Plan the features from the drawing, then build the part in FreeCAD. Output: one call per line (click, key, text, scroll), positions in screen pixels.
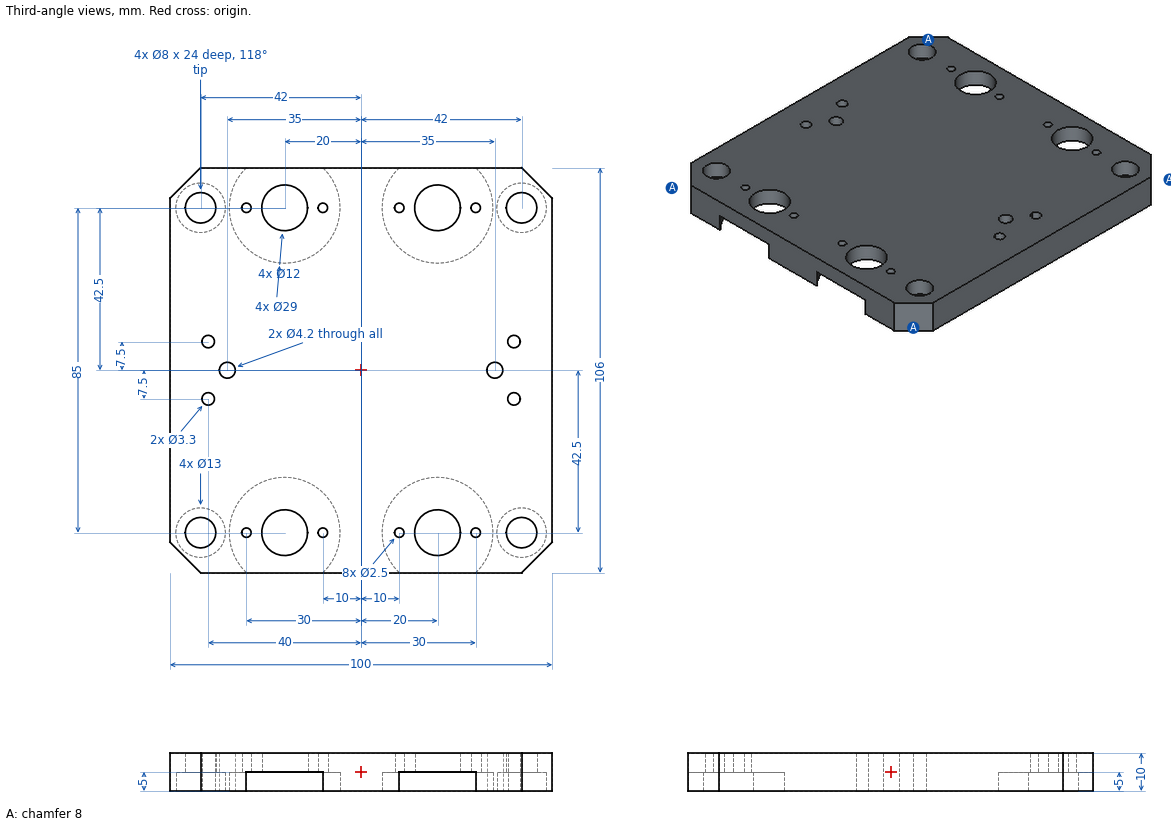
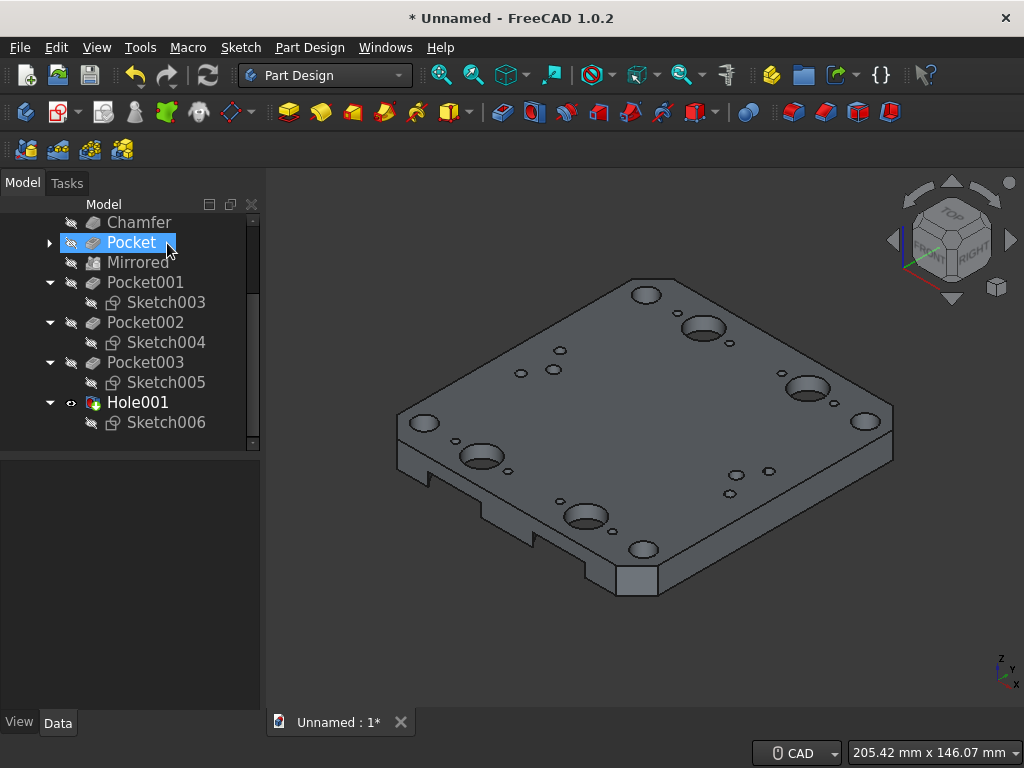
key(5)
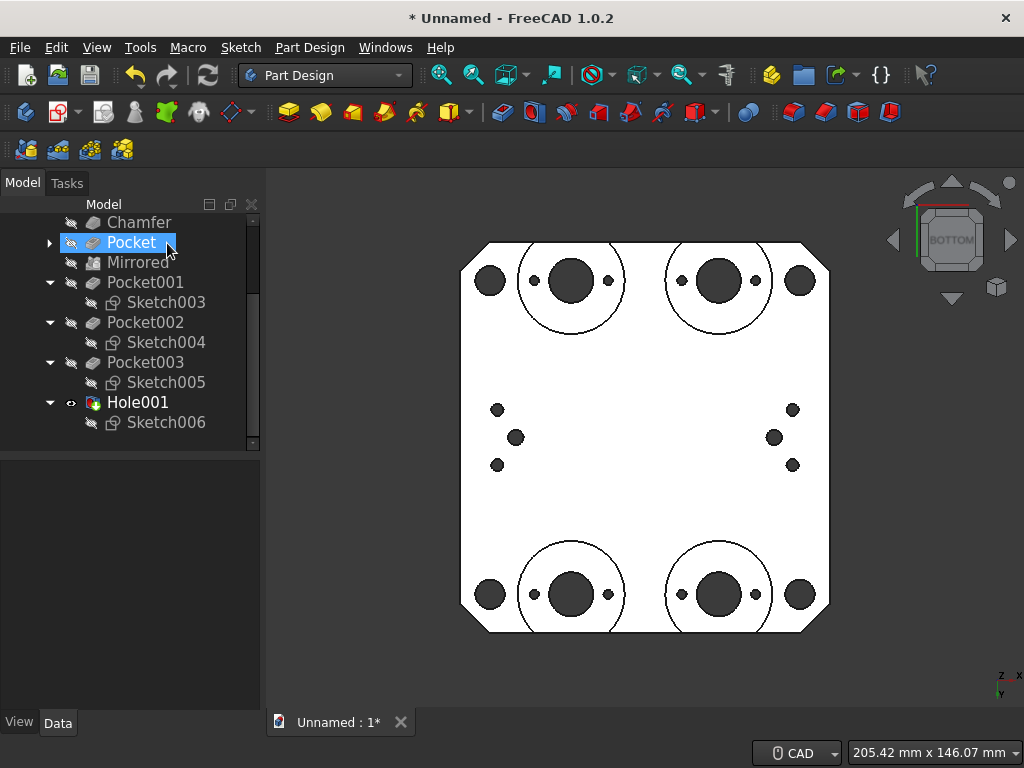
click(645, 437)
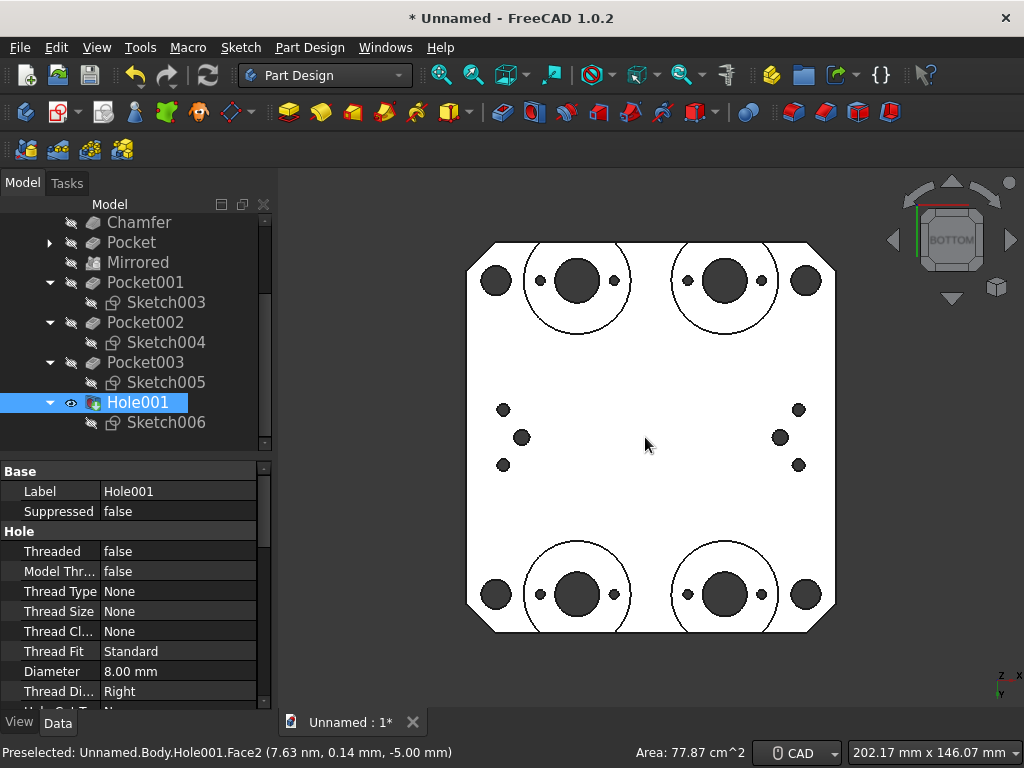
click(58, 112)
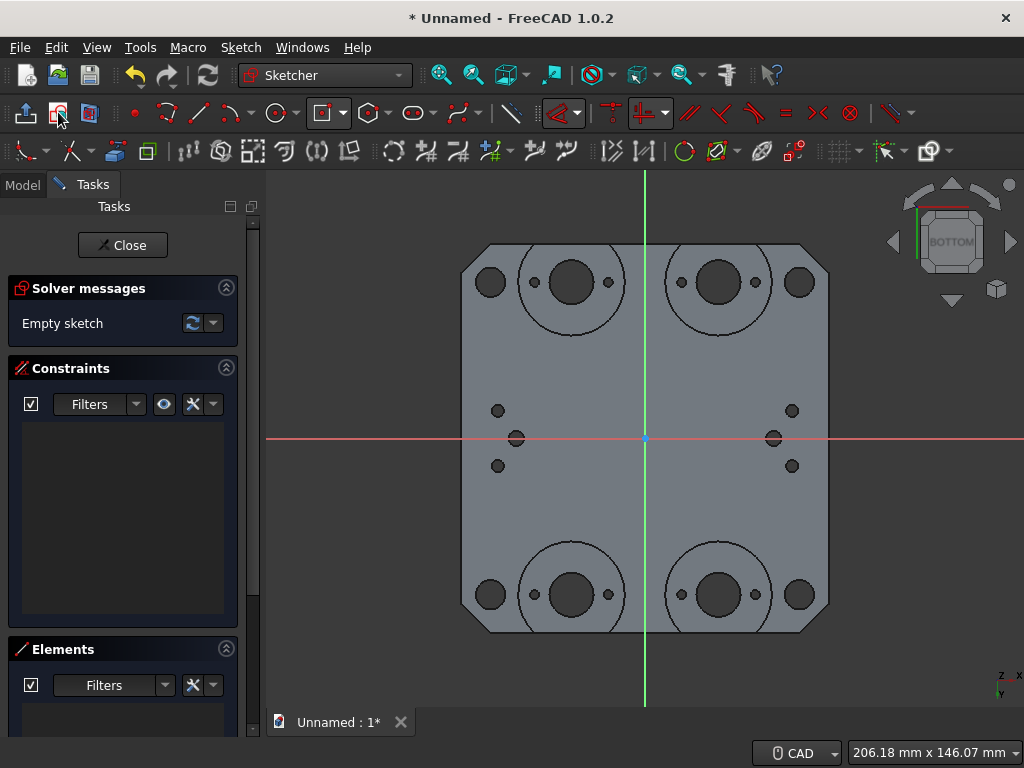
click(276, 114)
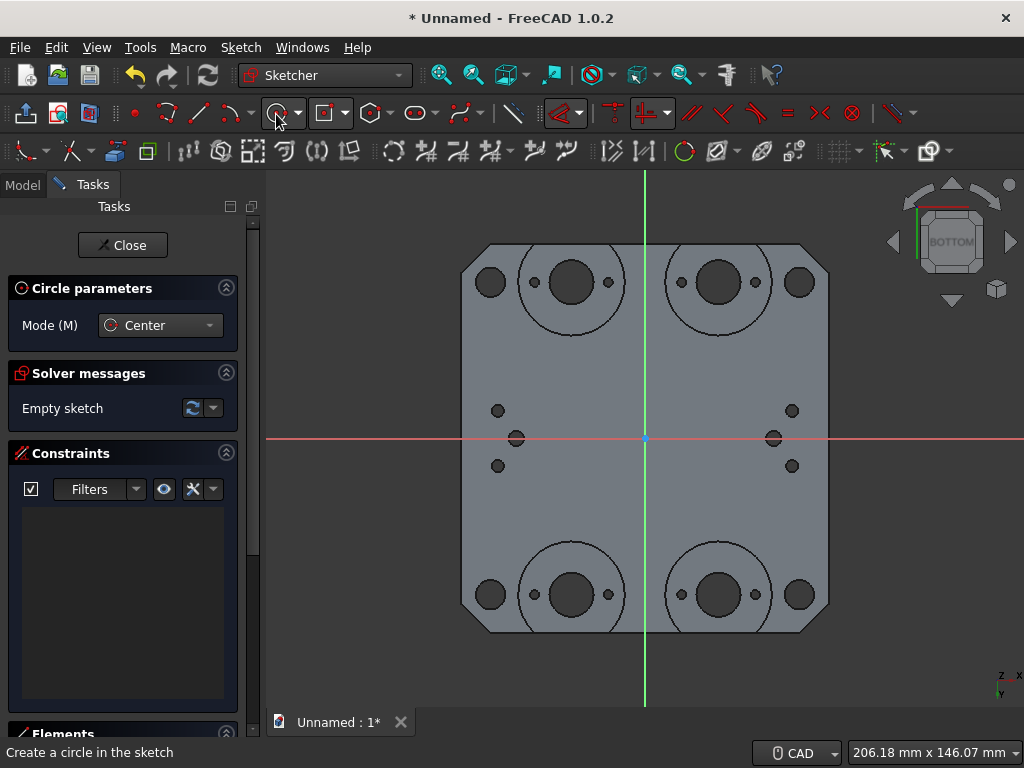
click(491, 282)
move(507, 265)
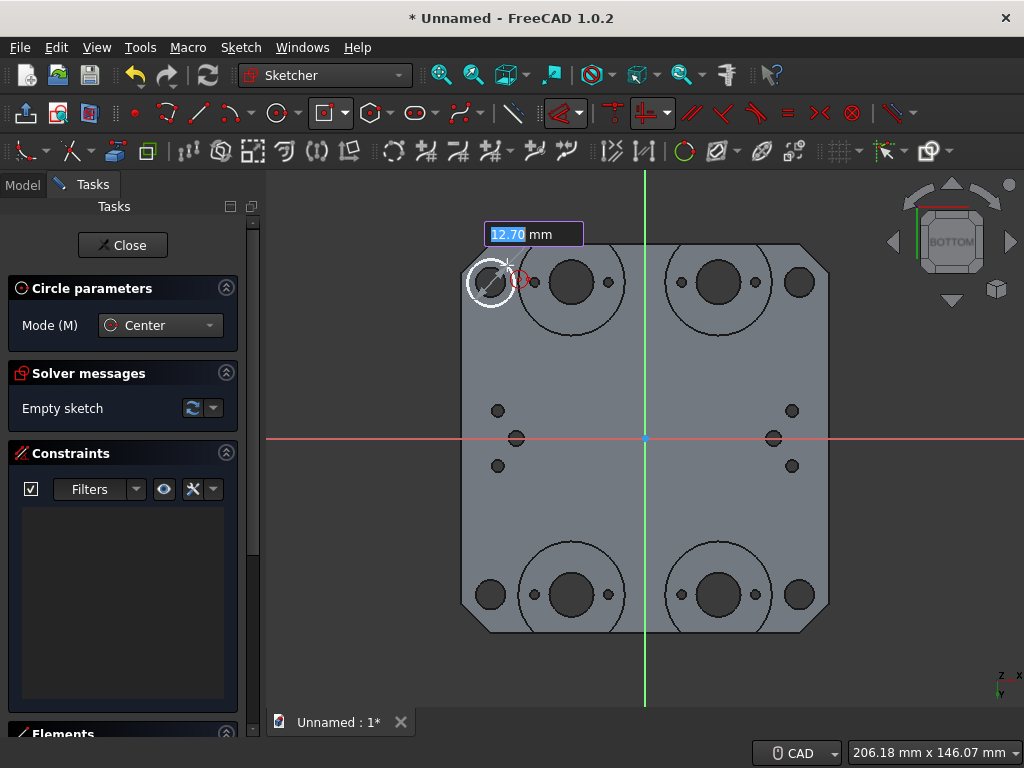
text(13)
key(Return)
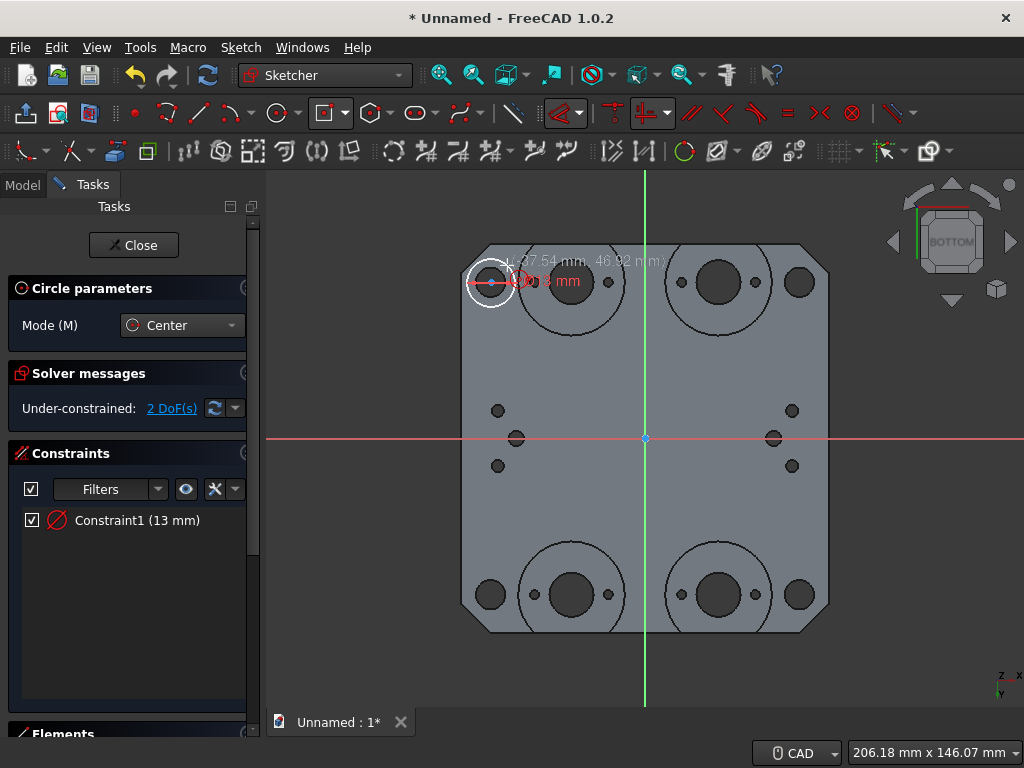
click(799, 282)
move(816, 265)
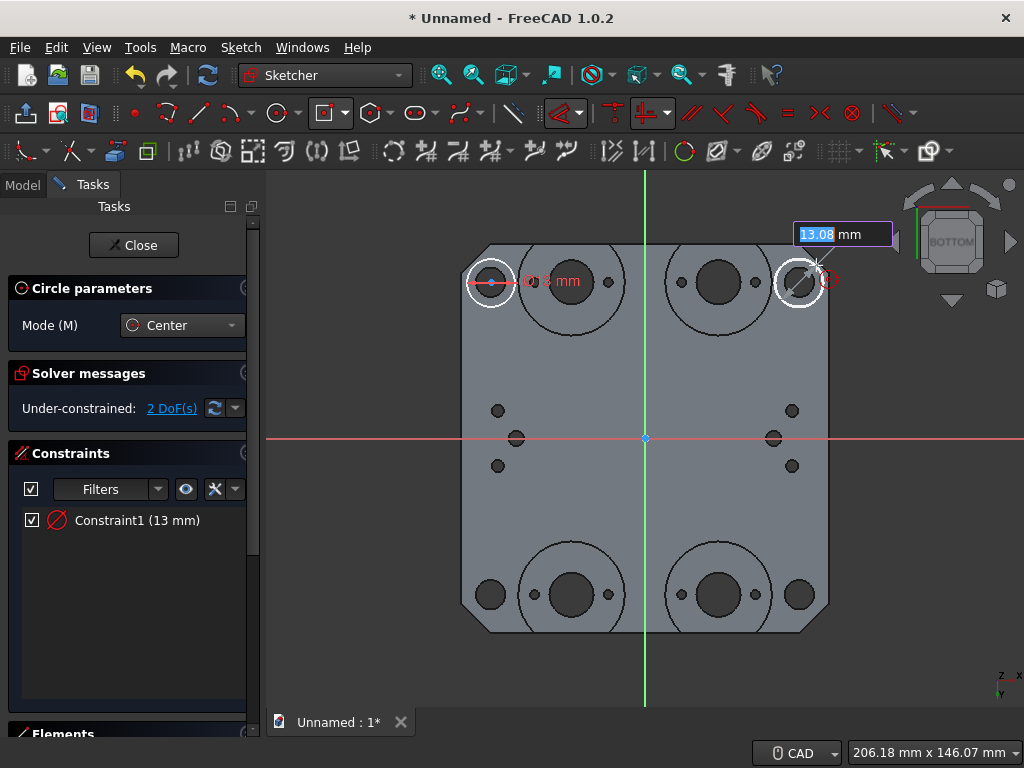
text(13)
key(Return)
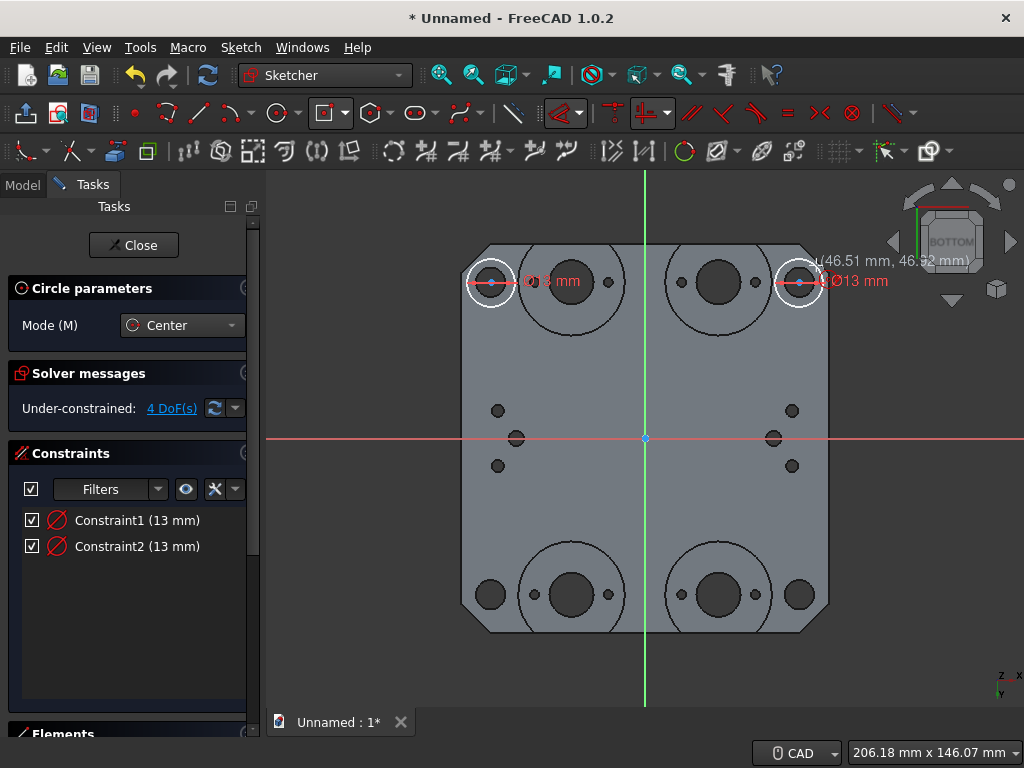
click(491, 595)
move(507, 578)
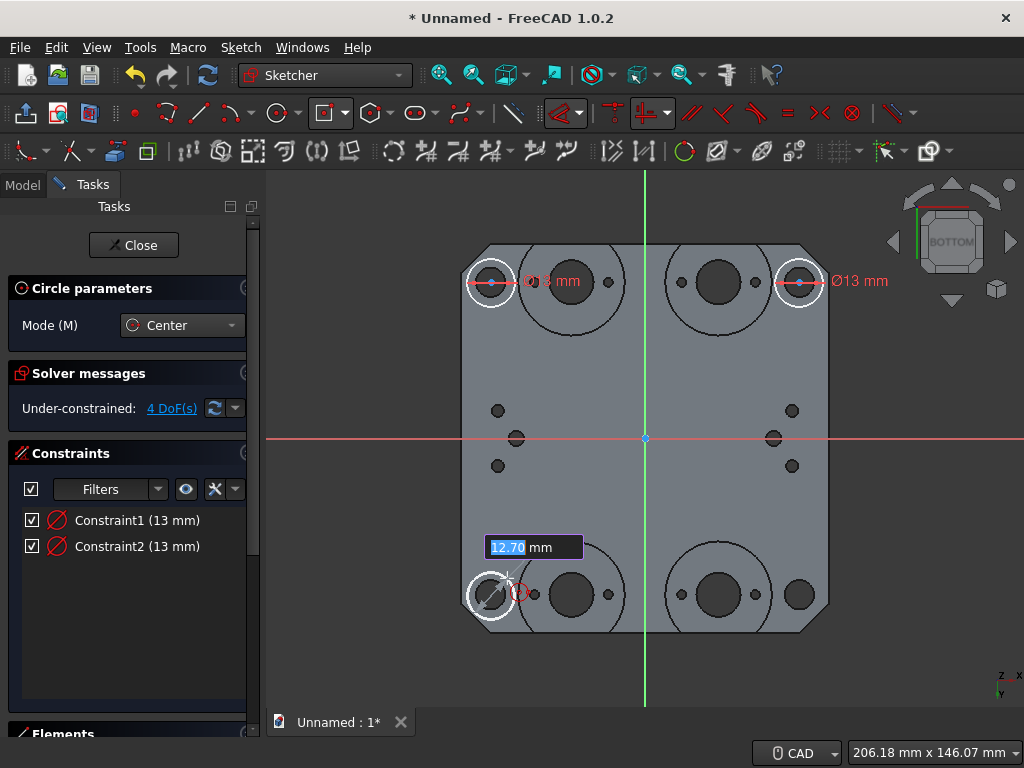
text(13)
key(Return)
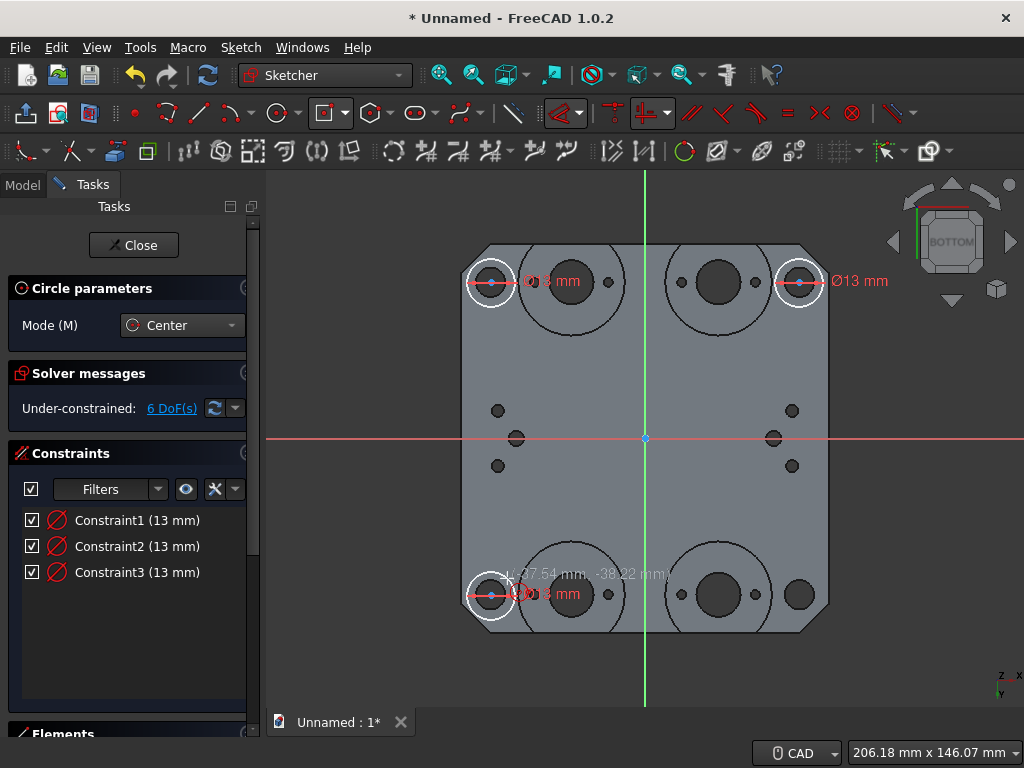
click(799, 595)
move(816, 578)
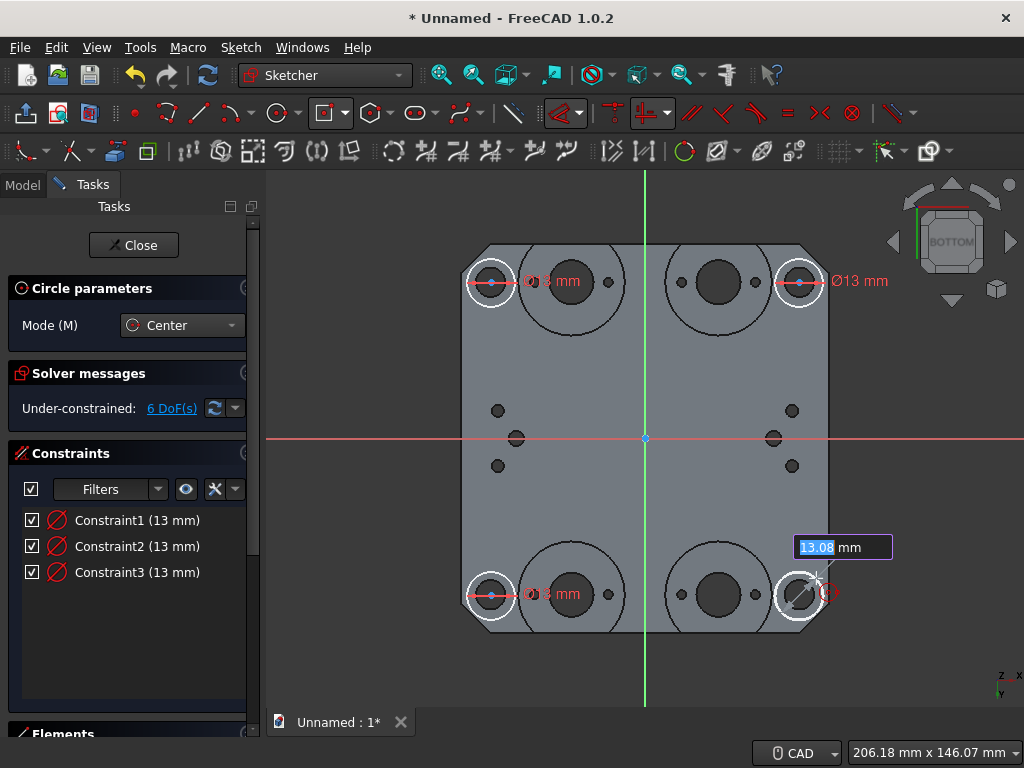
text(13)
key(Return)
key(Escape)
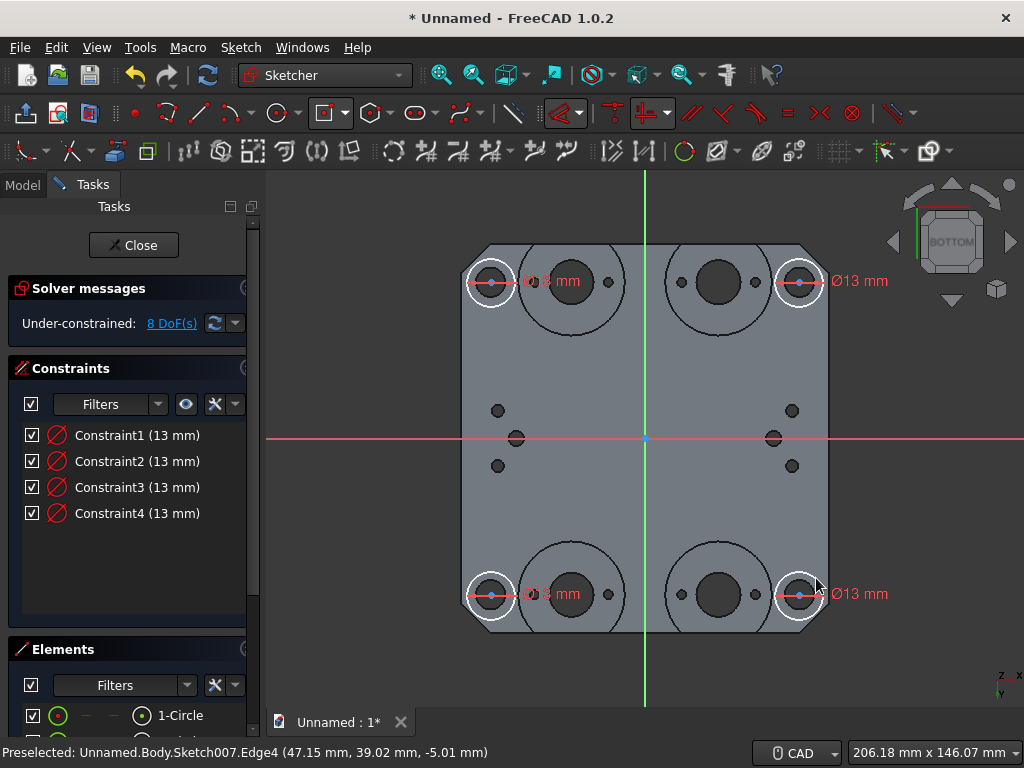
click(491, 283)